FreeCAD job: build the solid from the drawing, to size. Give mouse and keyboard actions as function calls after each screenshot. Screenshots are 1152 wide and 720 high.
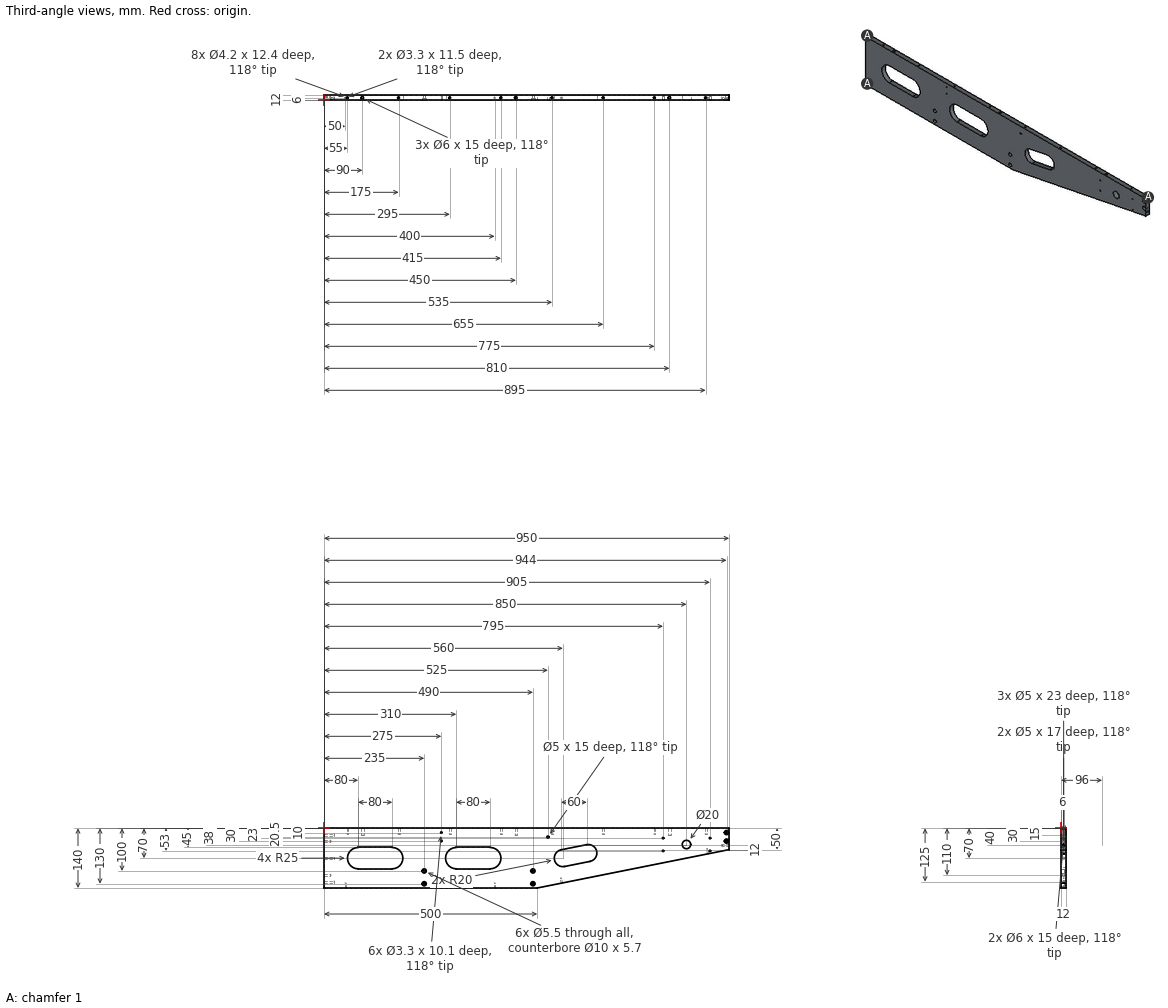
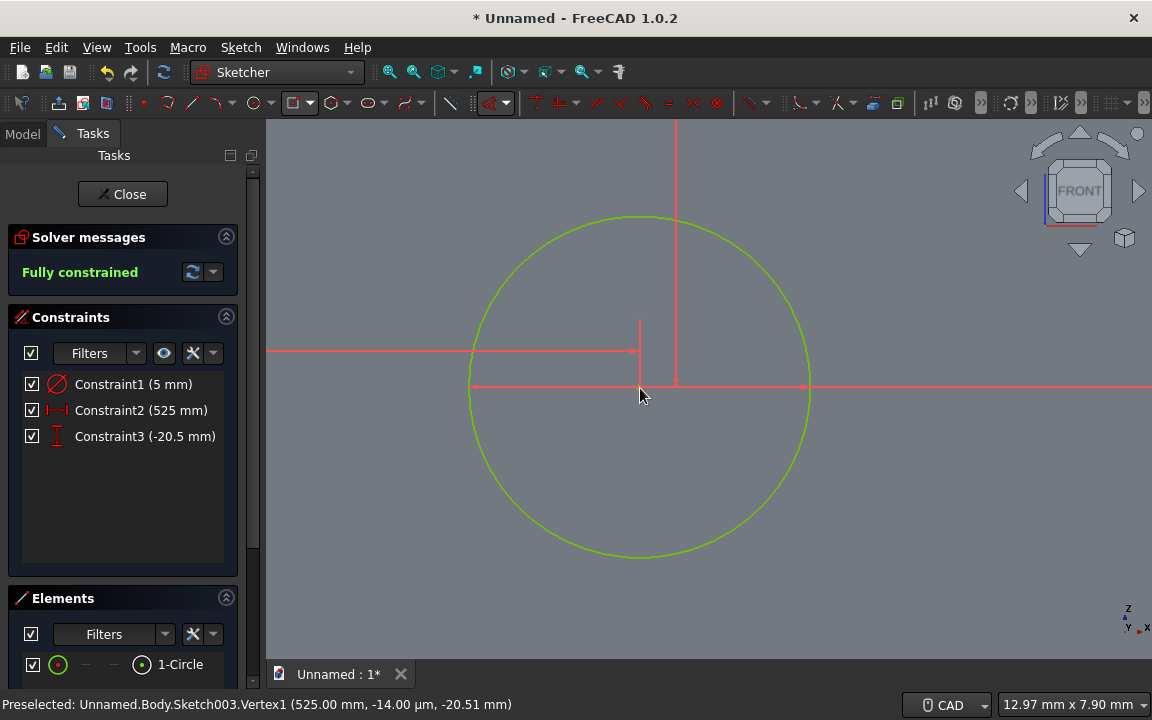
click(123, 194)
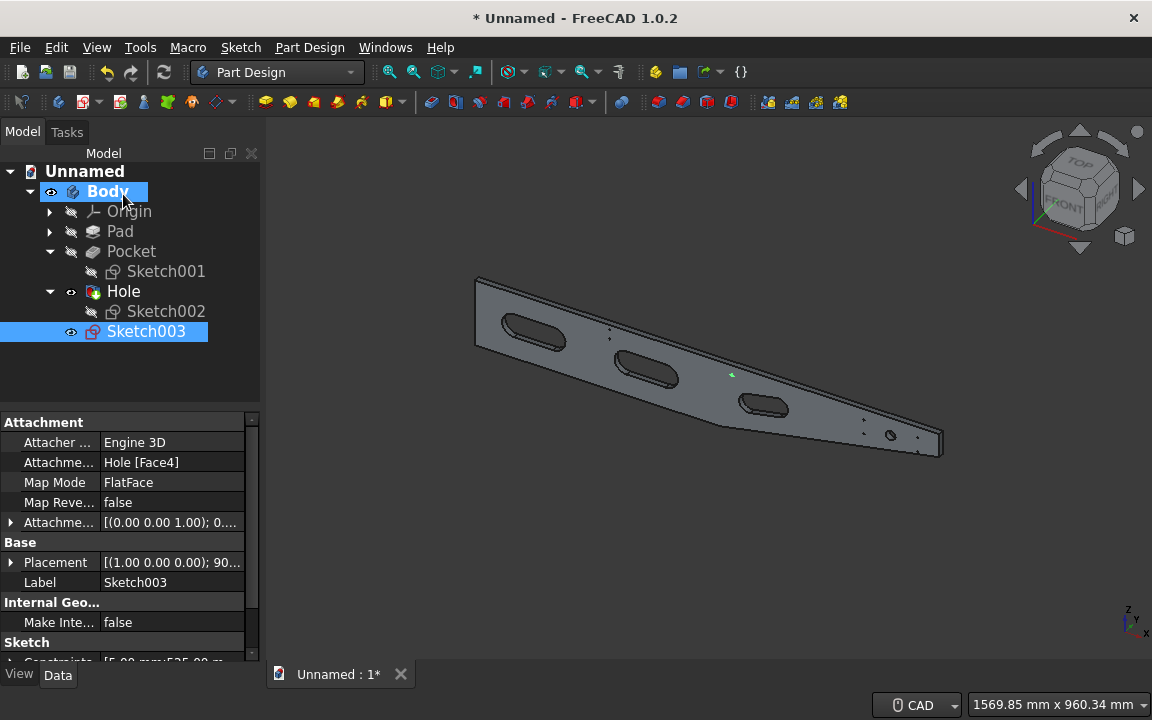
click(456, 102)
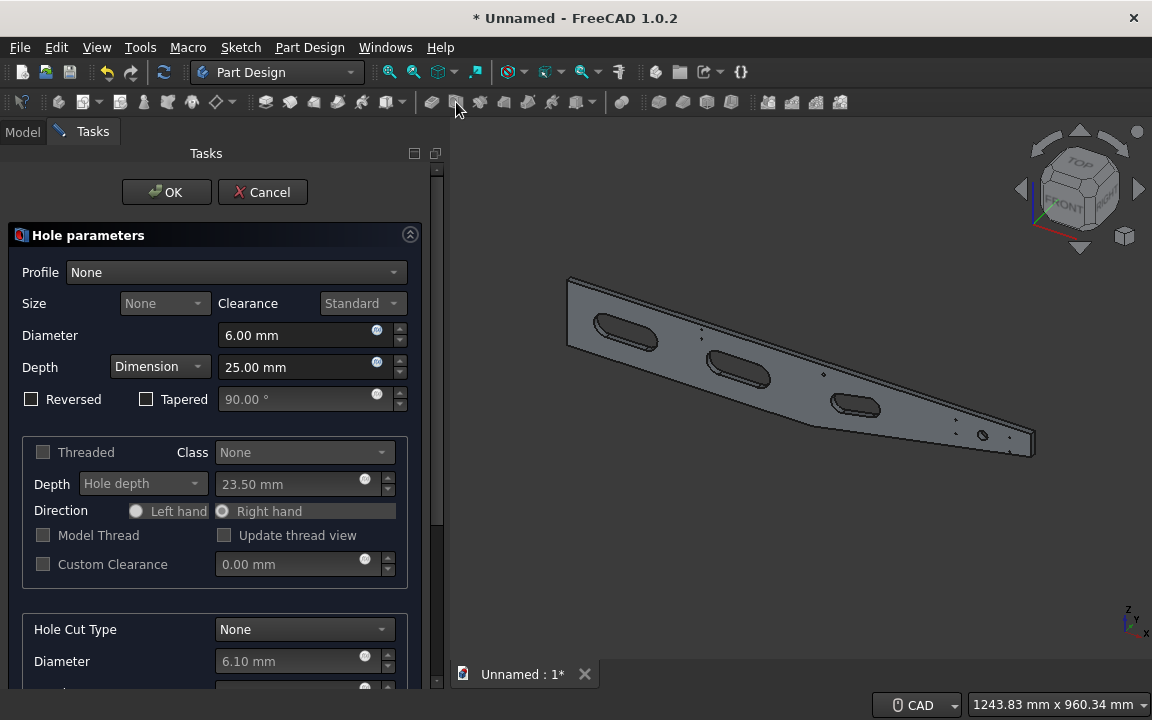
triple_click(305, 335)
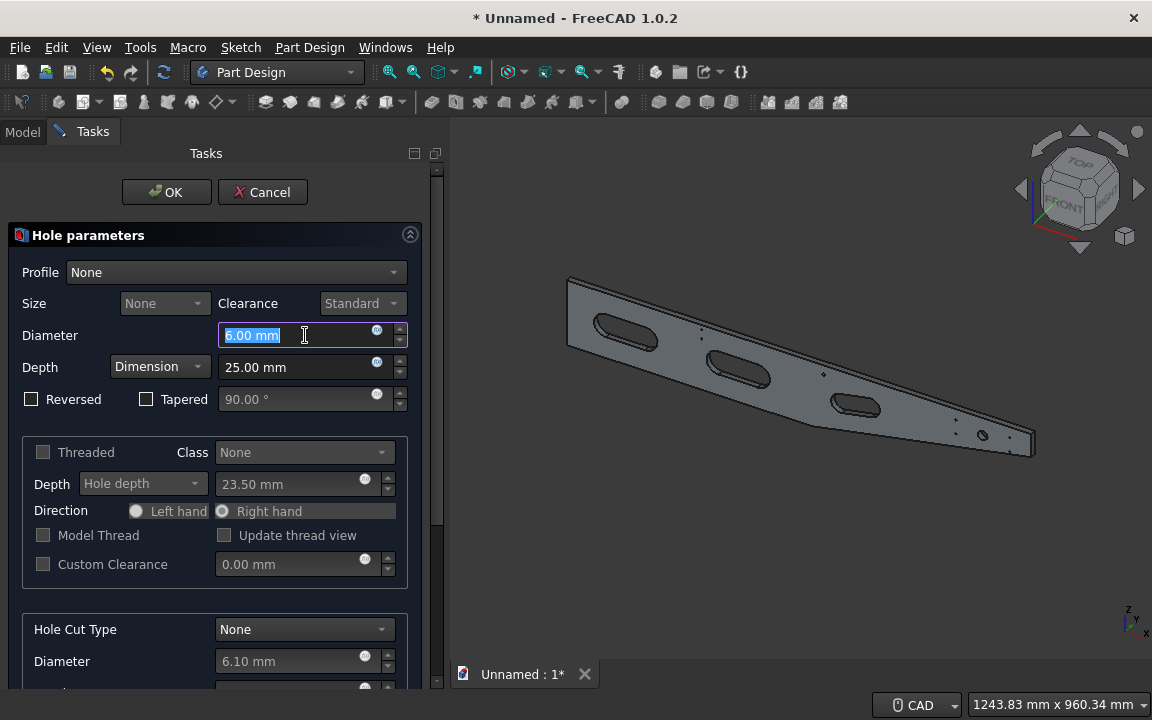
text(5)
key(Tab)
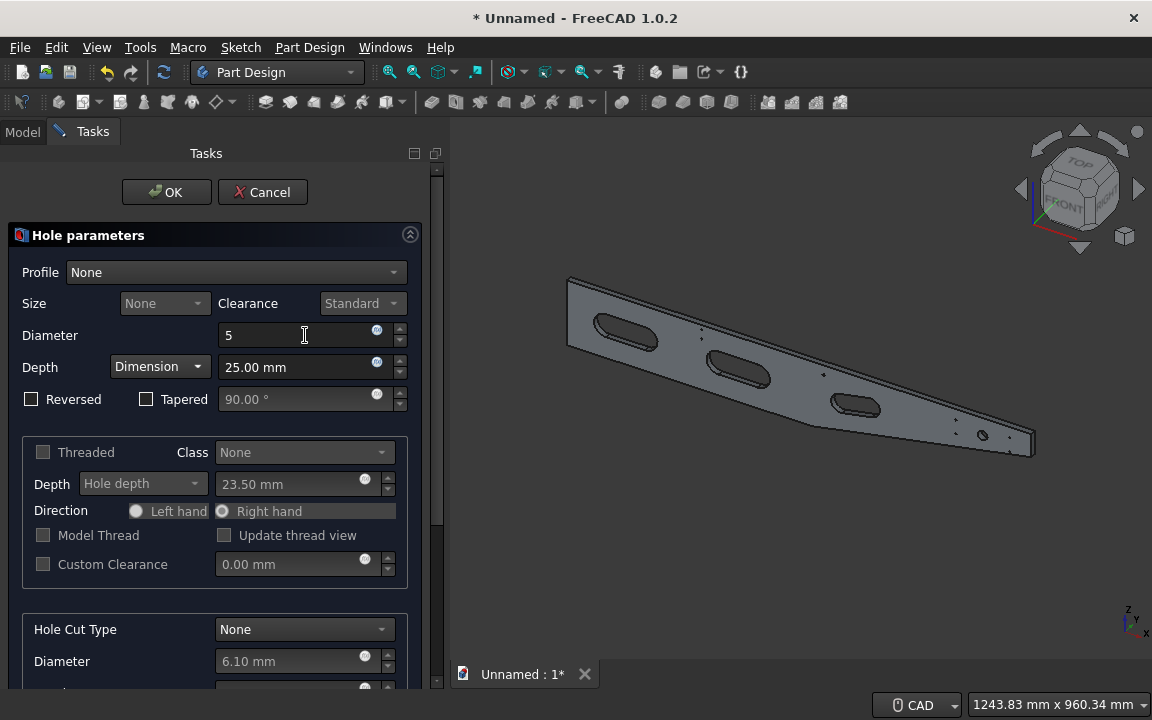
triple_click(305, 367)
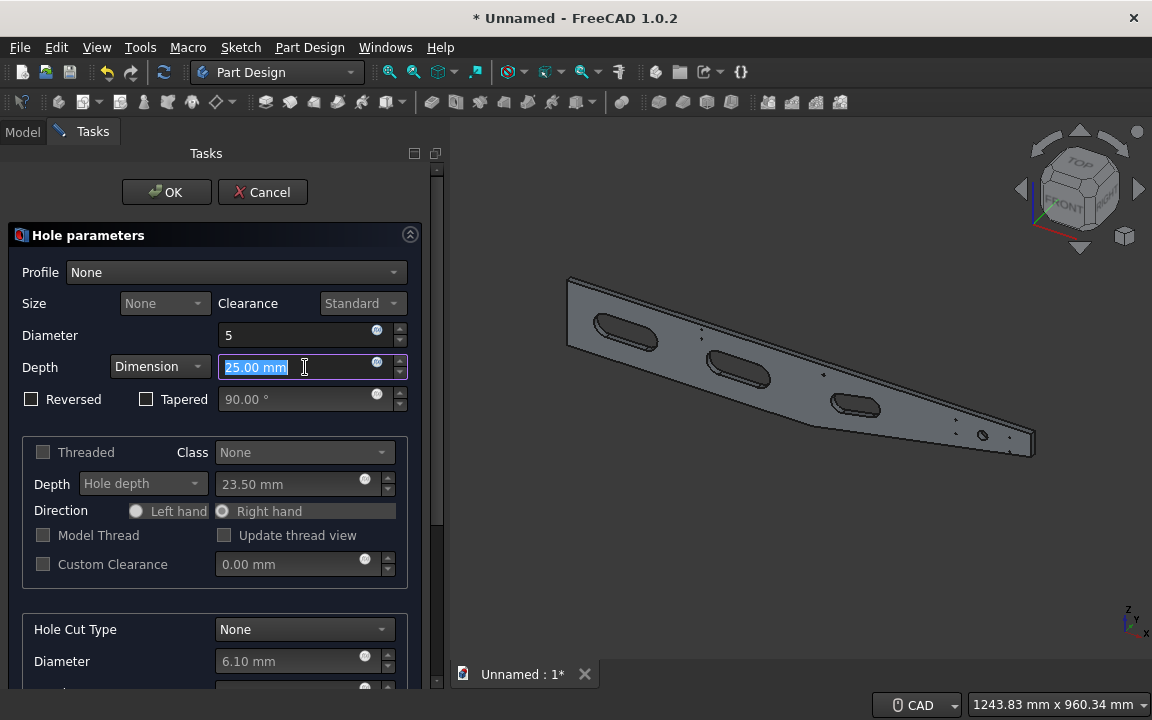
text(15)
key(Tab)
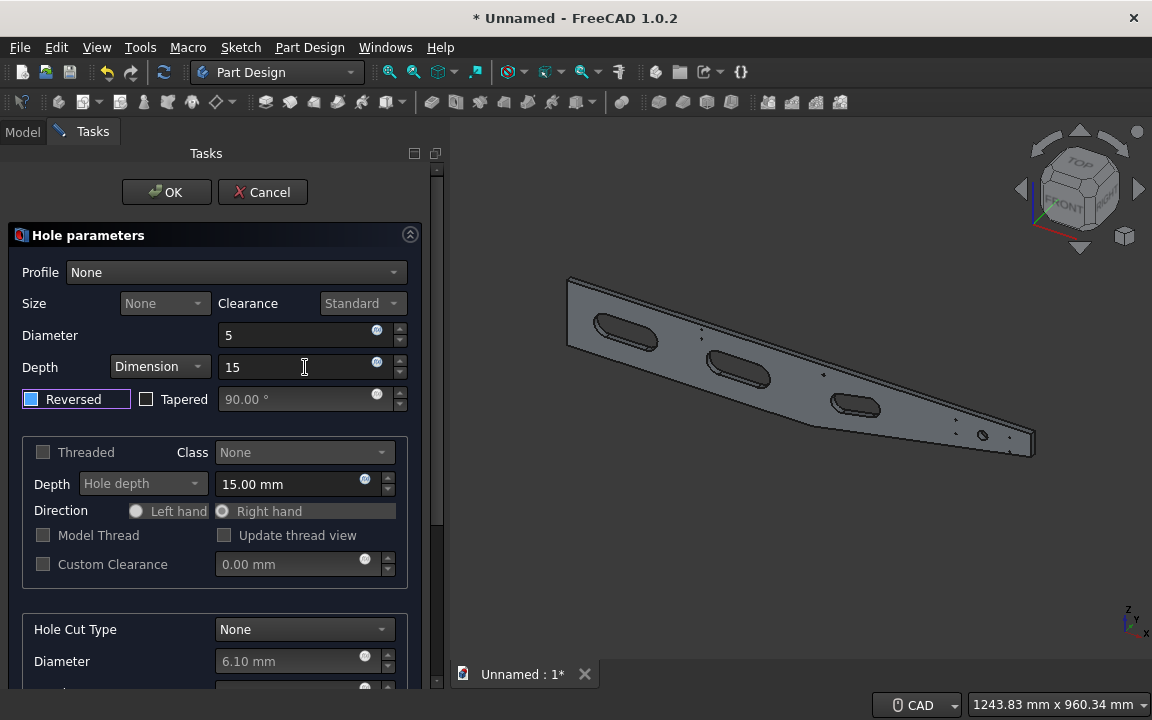
click(167, 192)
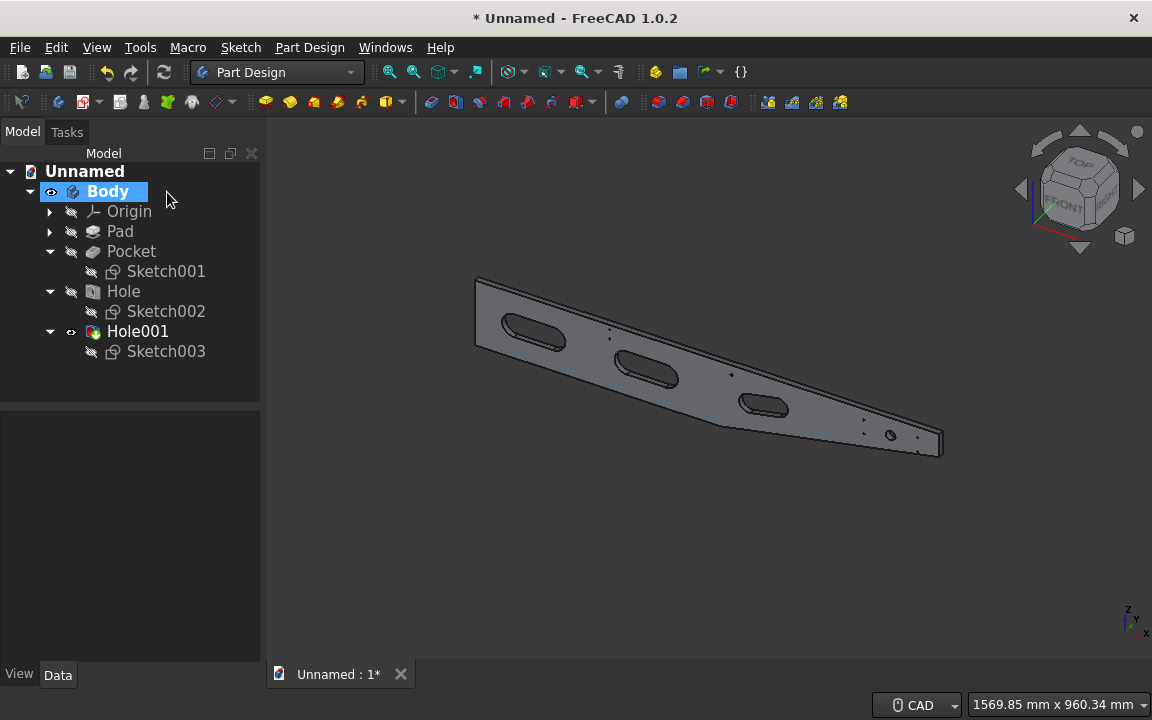
key(5)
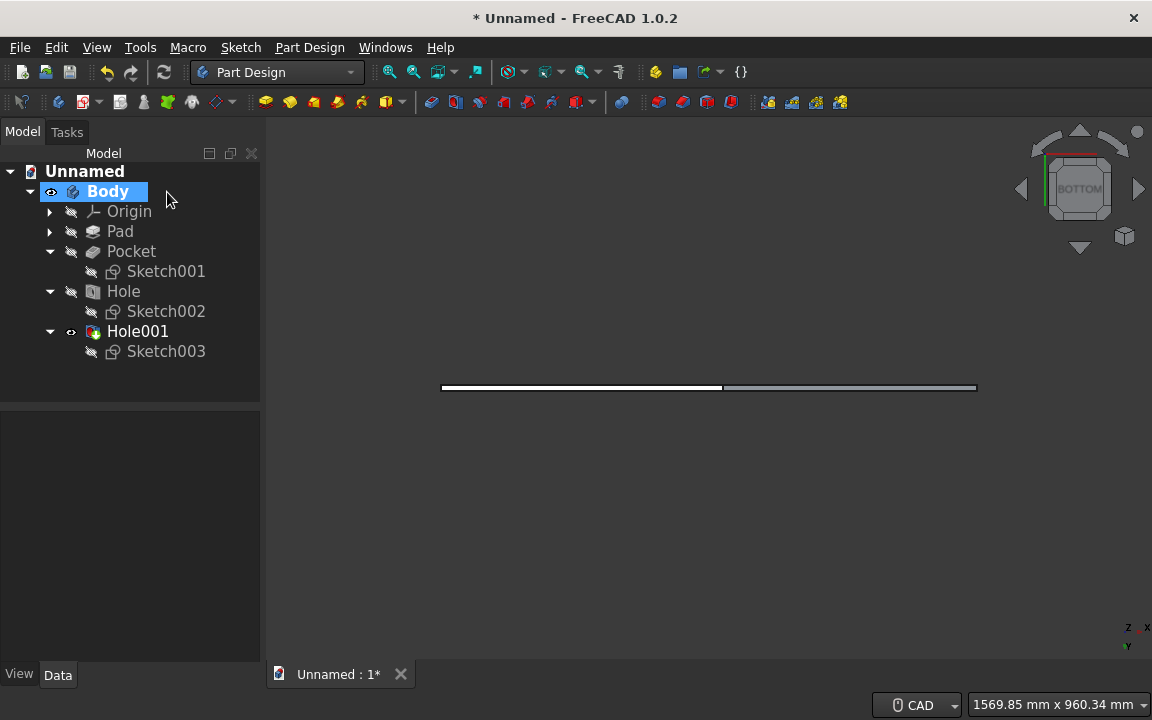
scroll(703, 387, up, 7)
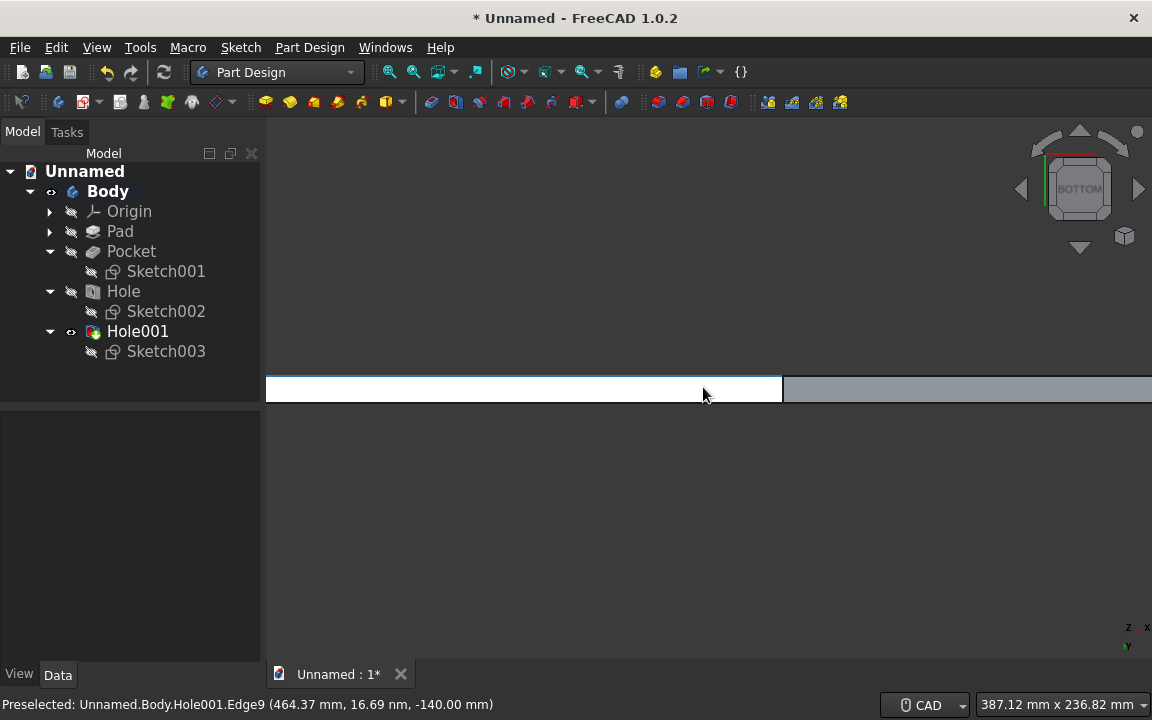
click(701, 389)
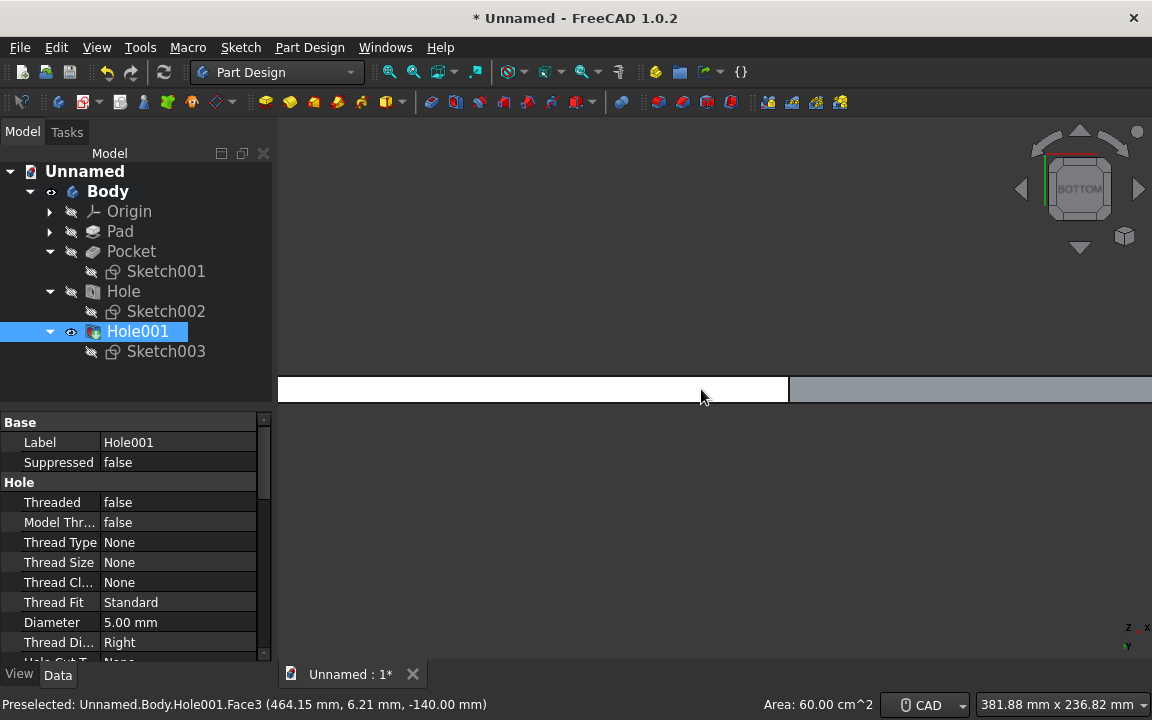
click(84, 102)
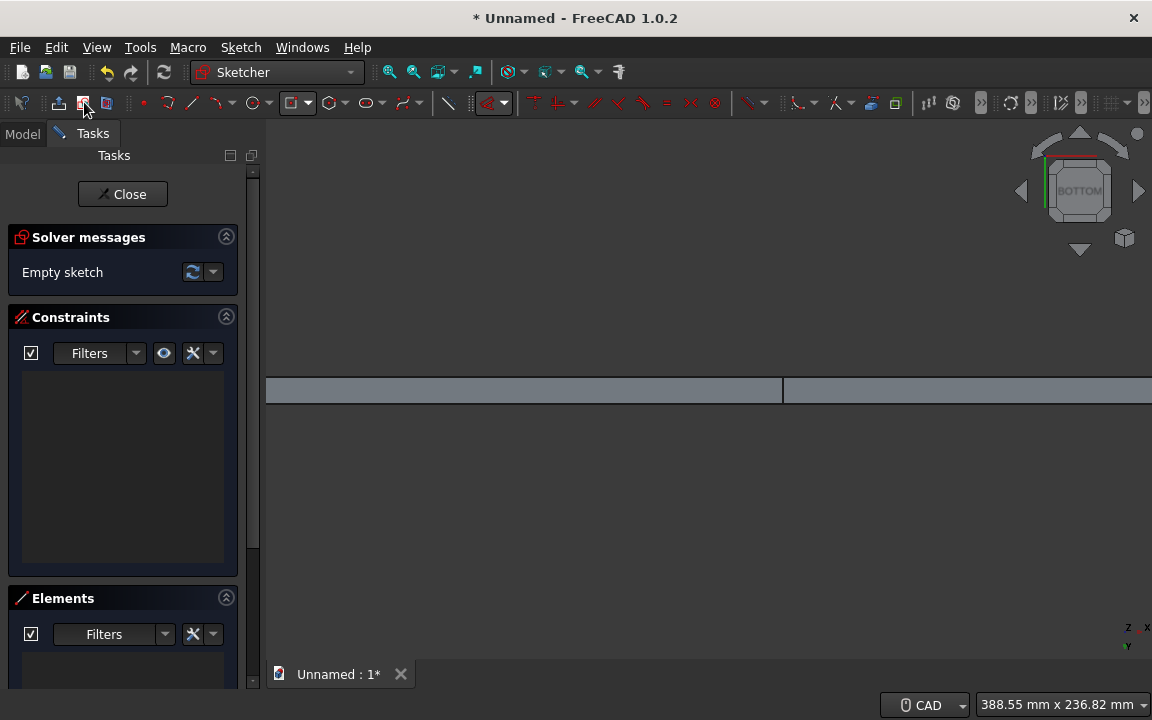
scroll(987, 392, down, 4)